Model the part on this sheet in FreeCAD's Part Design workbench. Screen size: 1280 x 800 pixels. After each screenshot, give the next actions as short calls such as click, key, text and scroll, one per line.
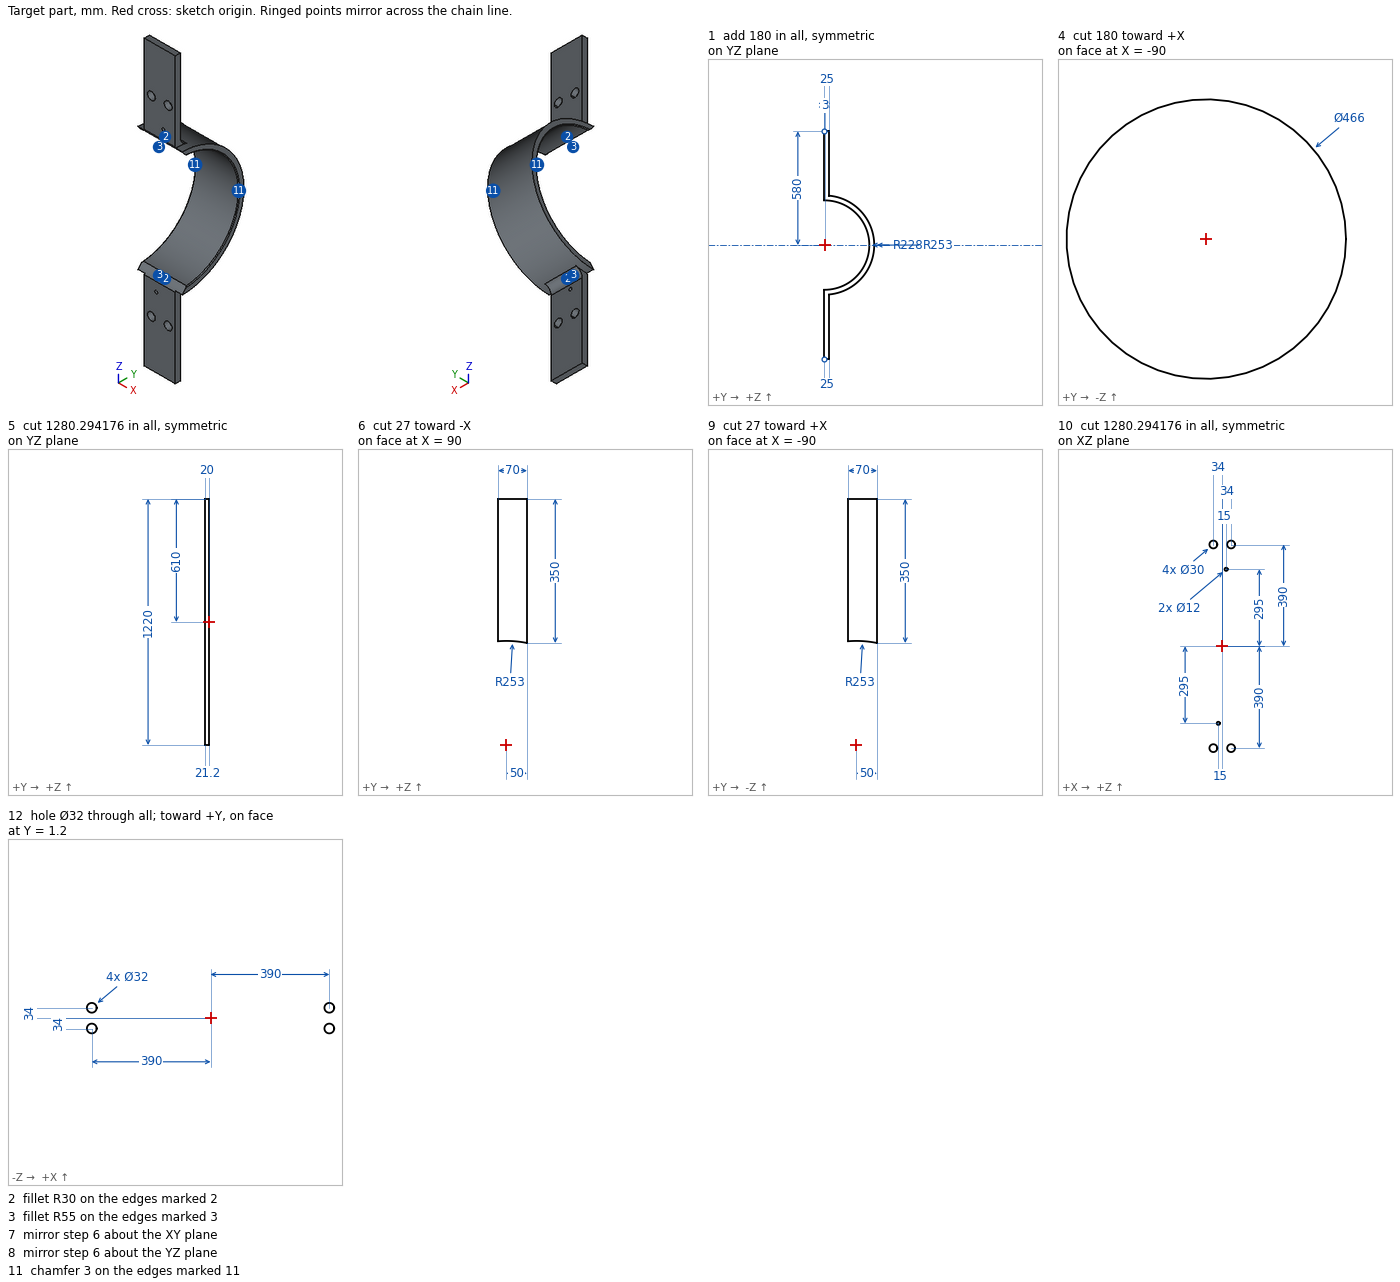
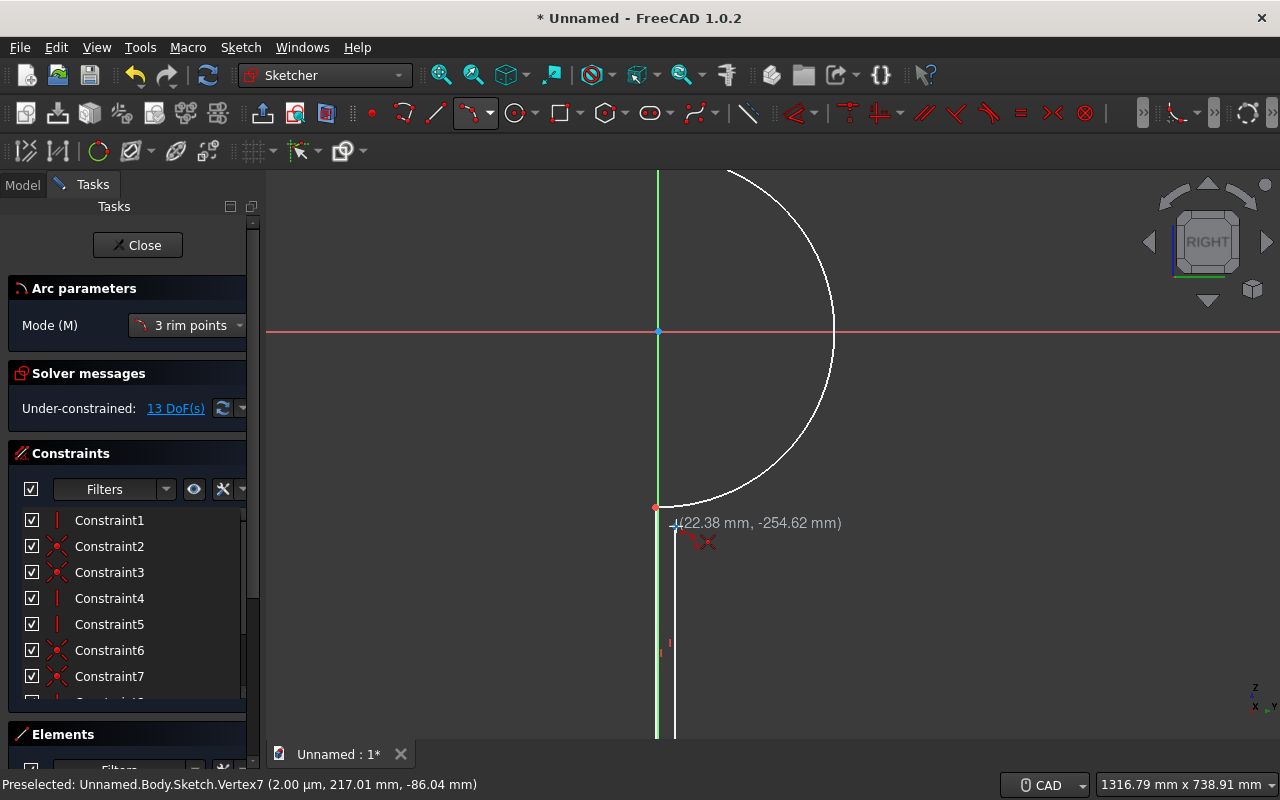
click(675, 526)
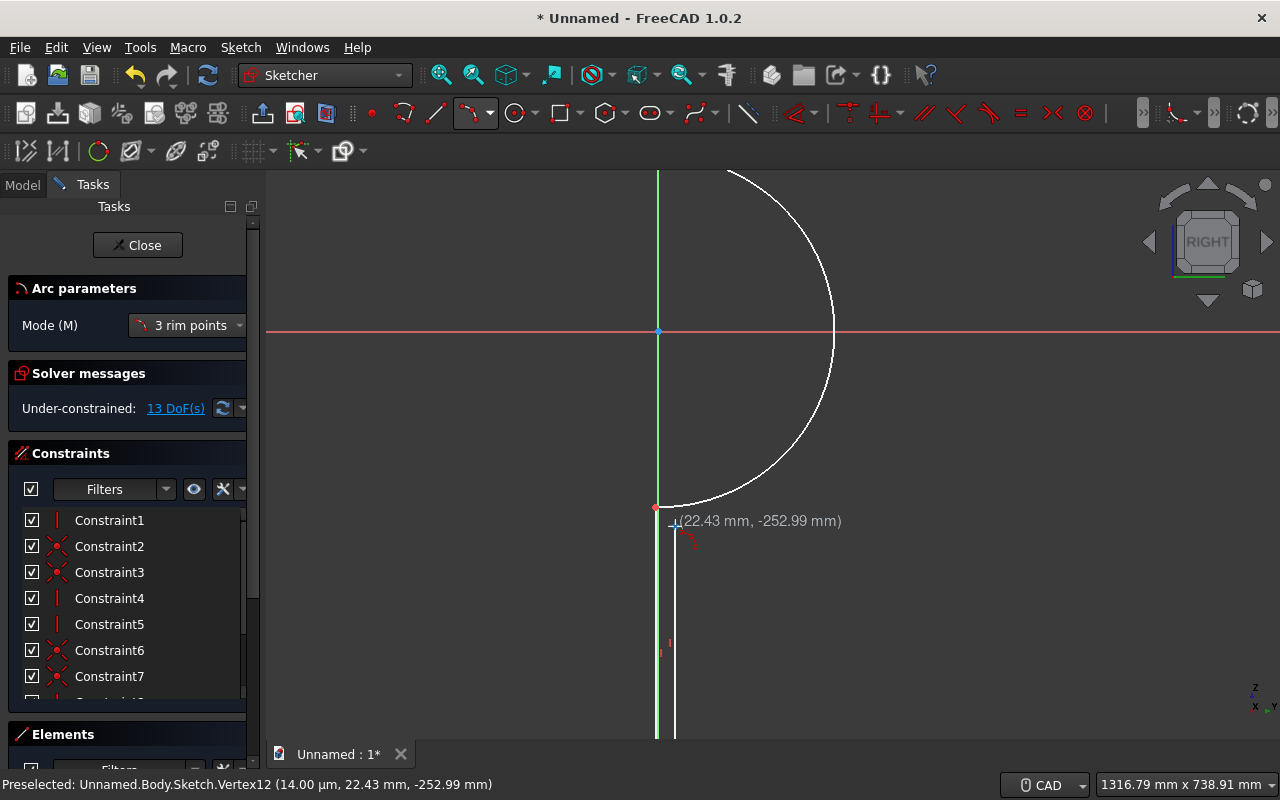
scroll(676, 526, down, 5)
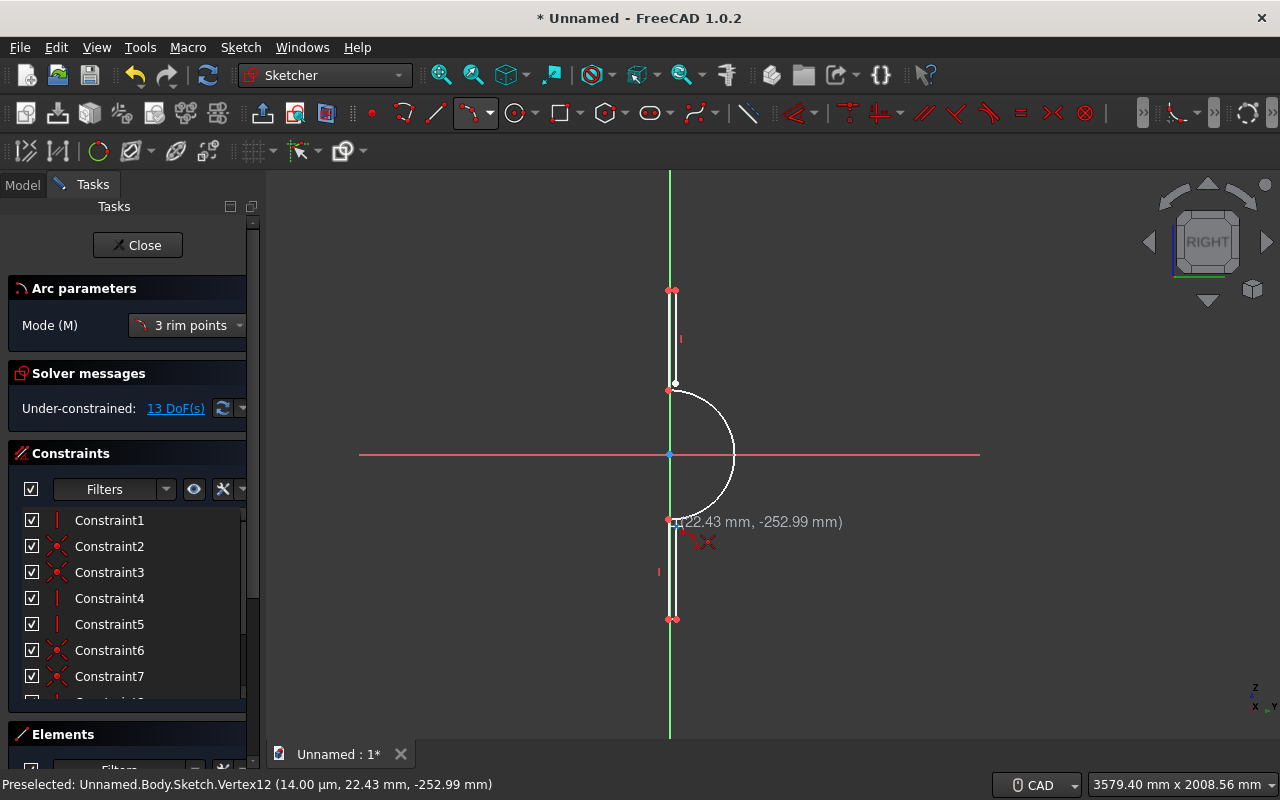
scroll(676, 383, up, 5)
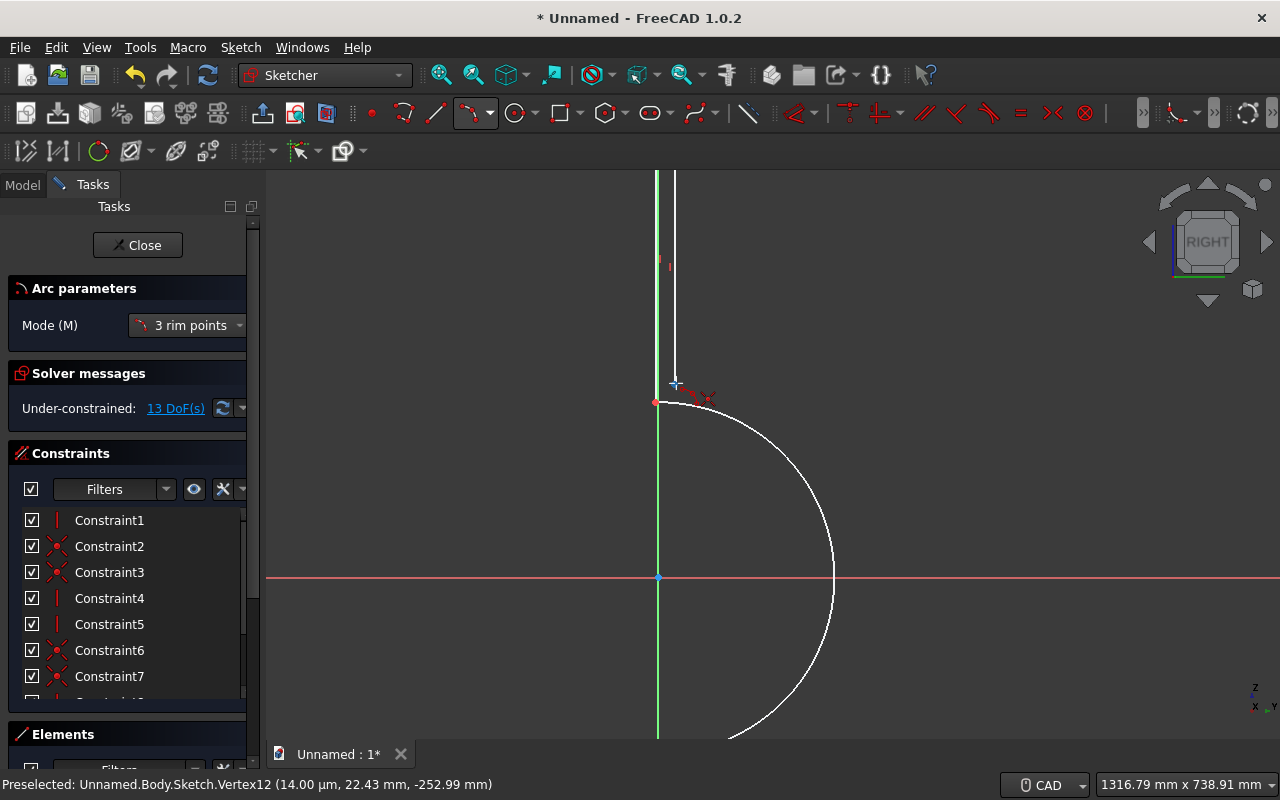
click(675, 385)
click(844, 635)
key(Escape)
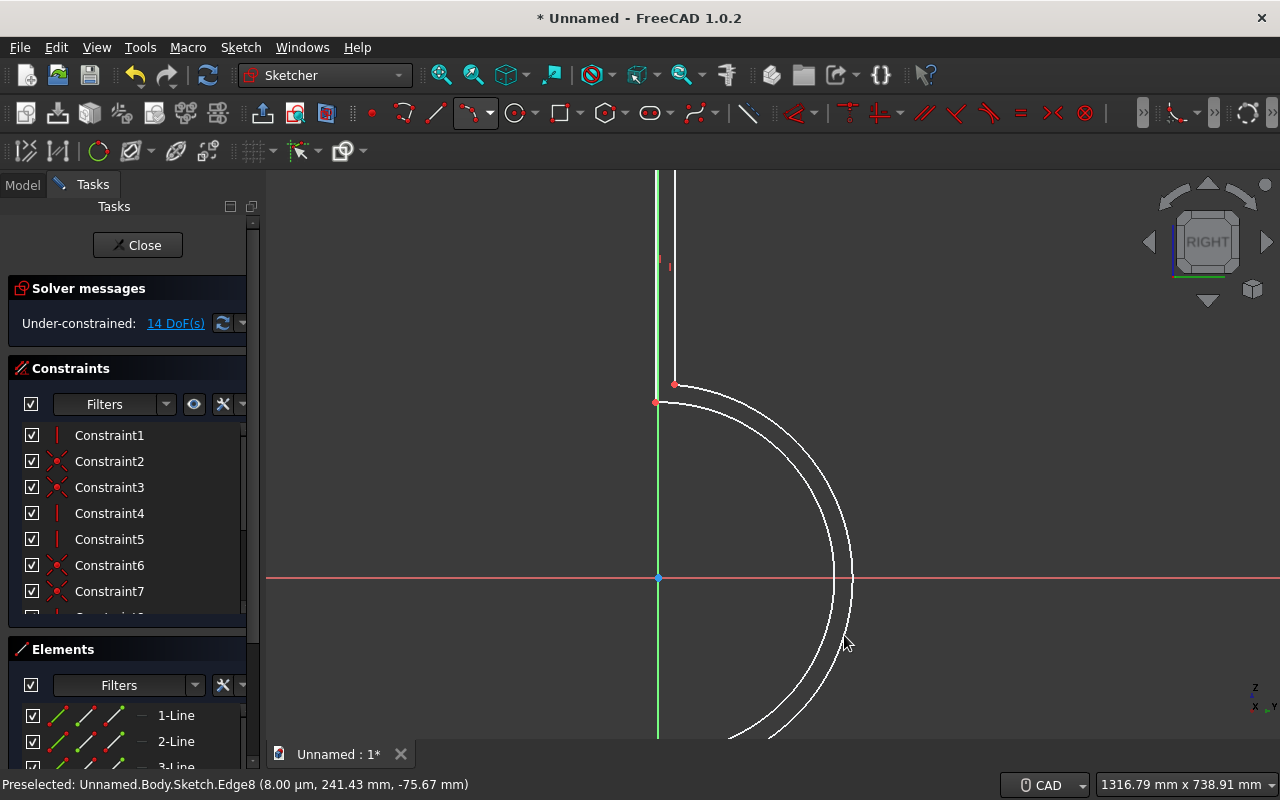
scroll(676, 383, down, 5)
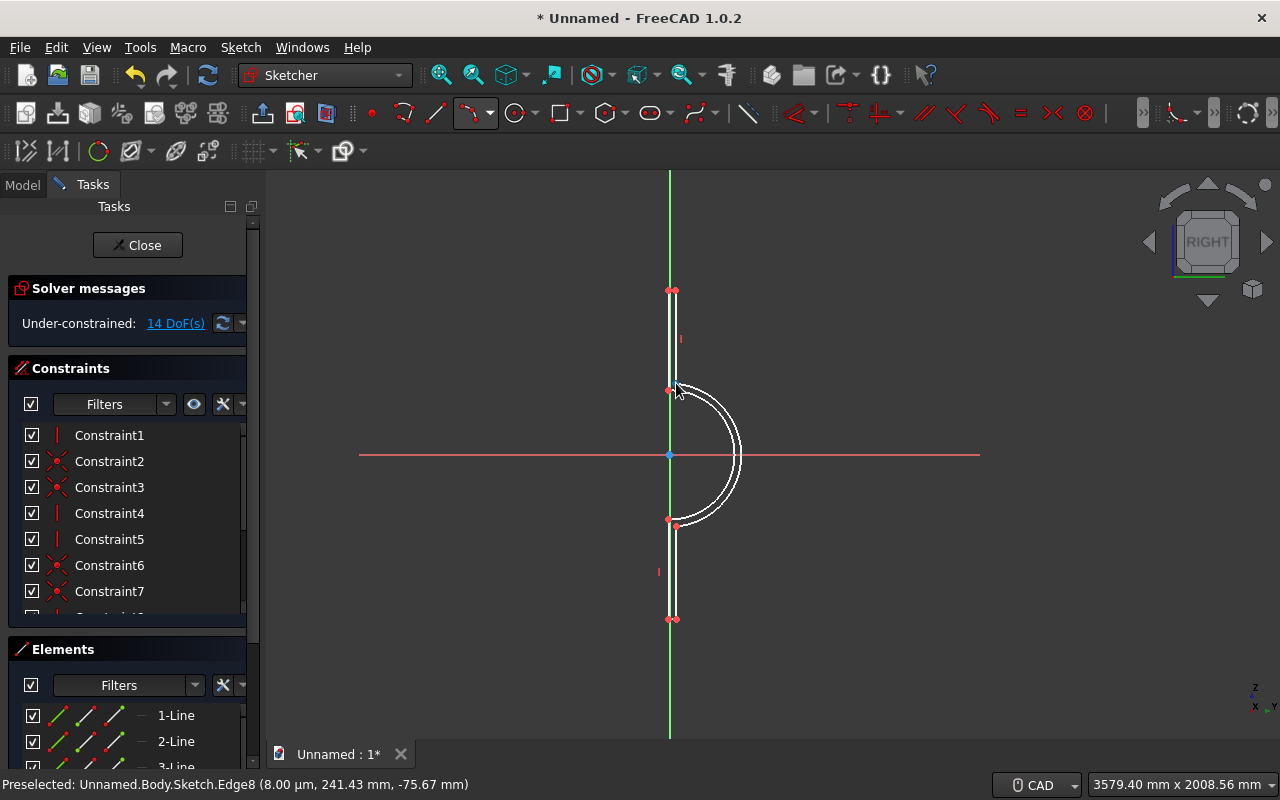
scroll(673, 291, up, 9)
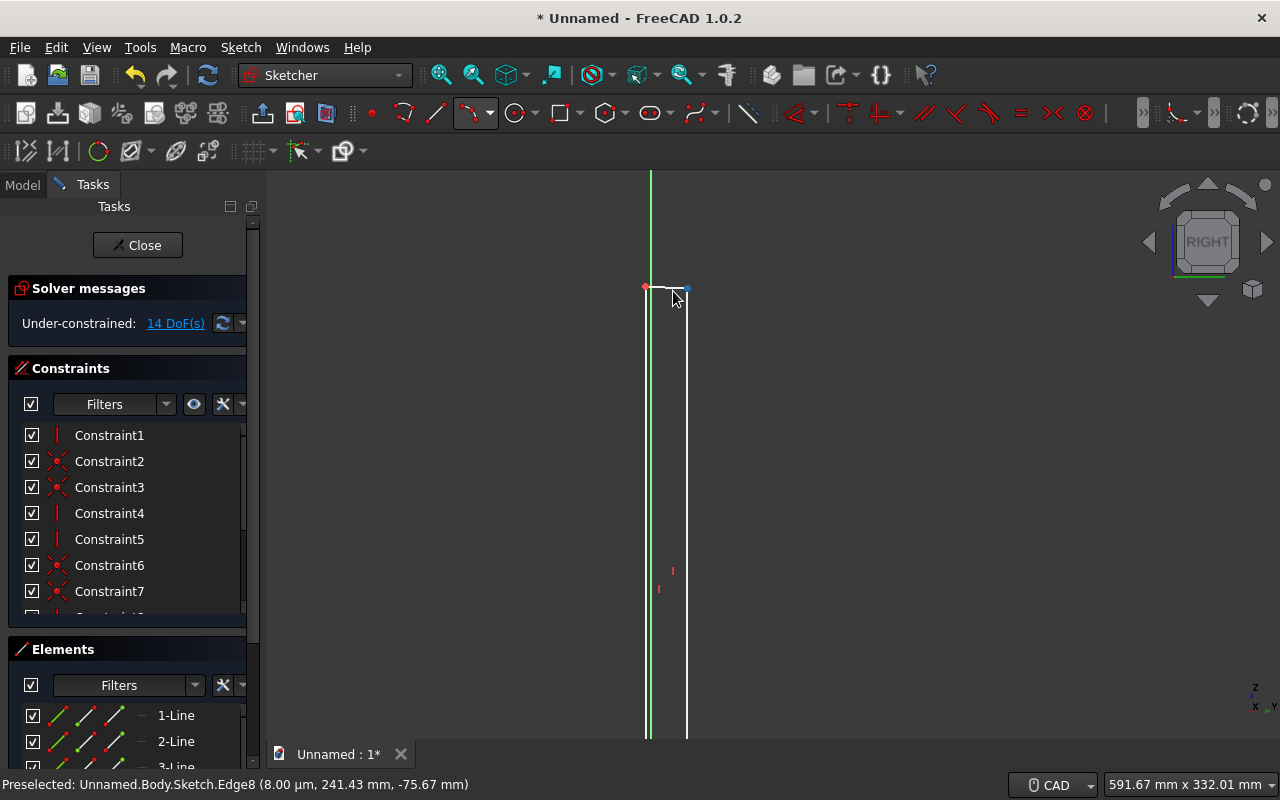
click(671, 288)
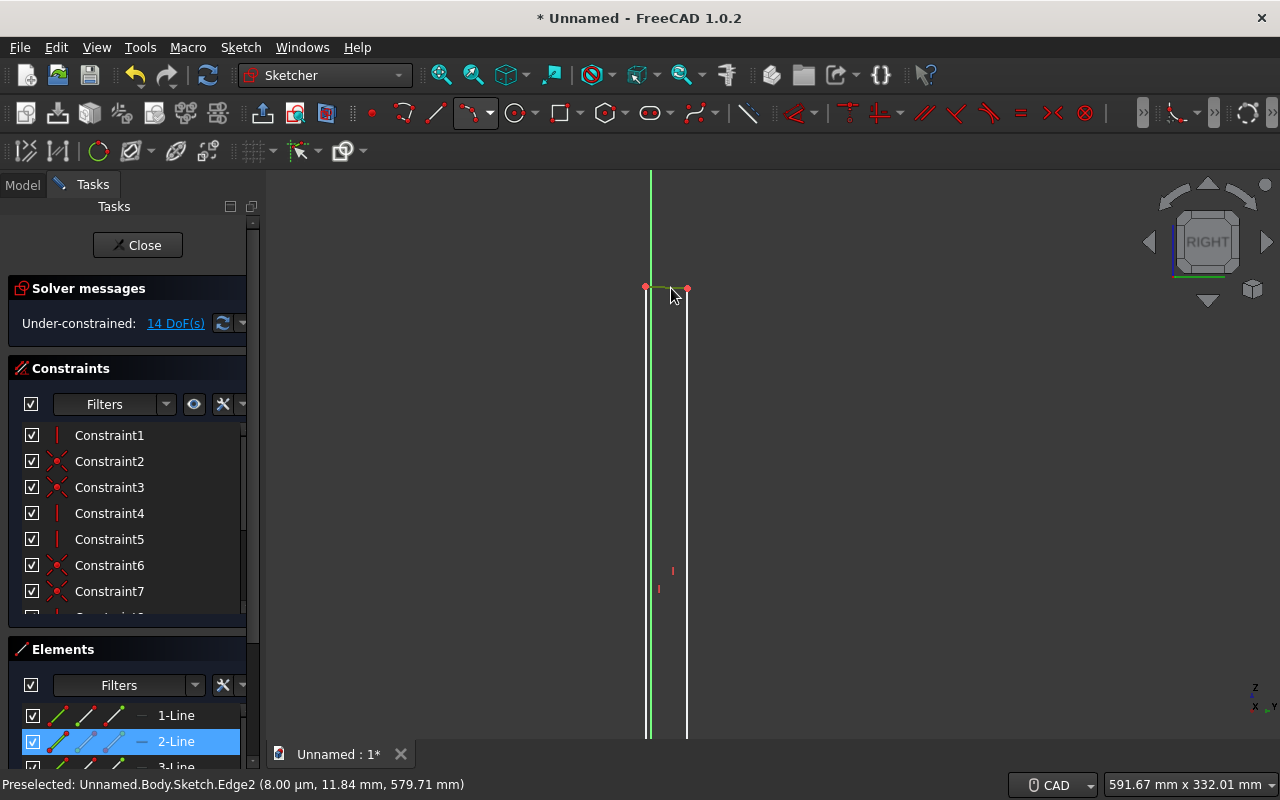
click(902, 114)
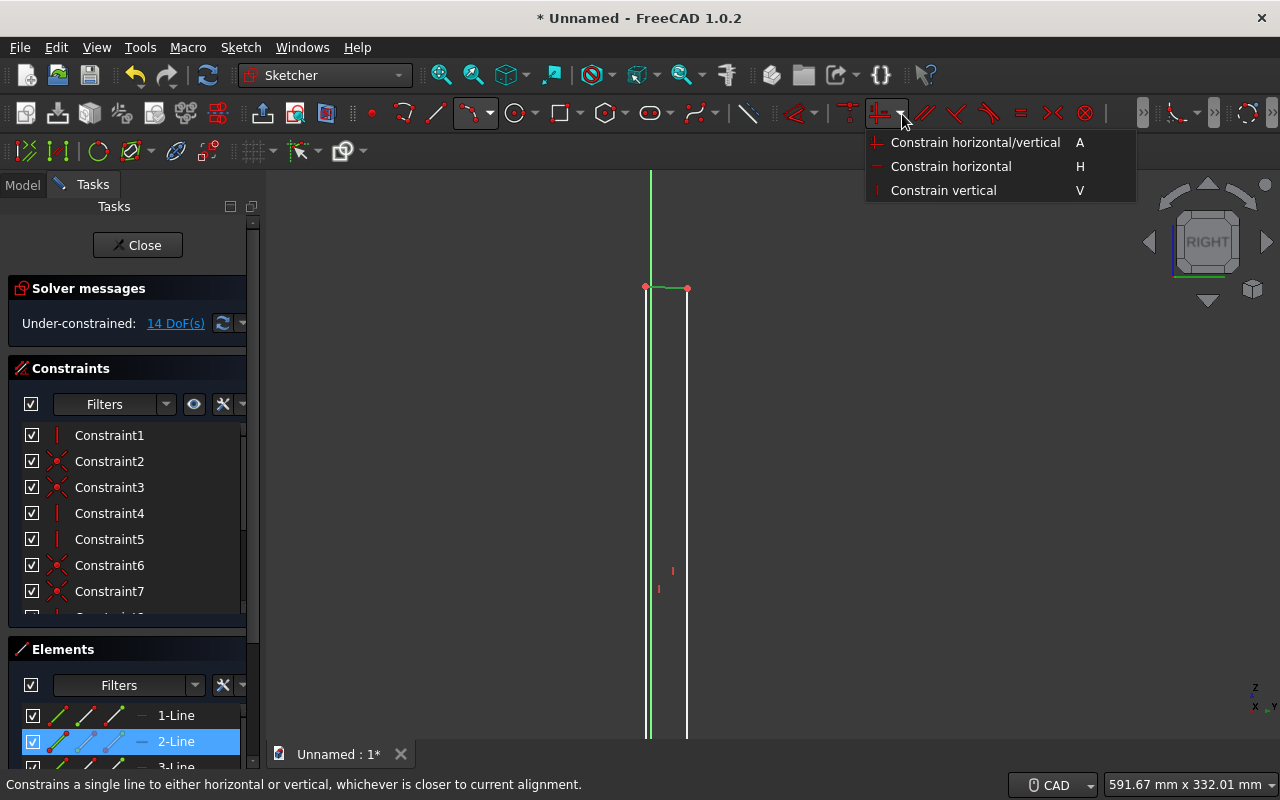
click(1001, 166)